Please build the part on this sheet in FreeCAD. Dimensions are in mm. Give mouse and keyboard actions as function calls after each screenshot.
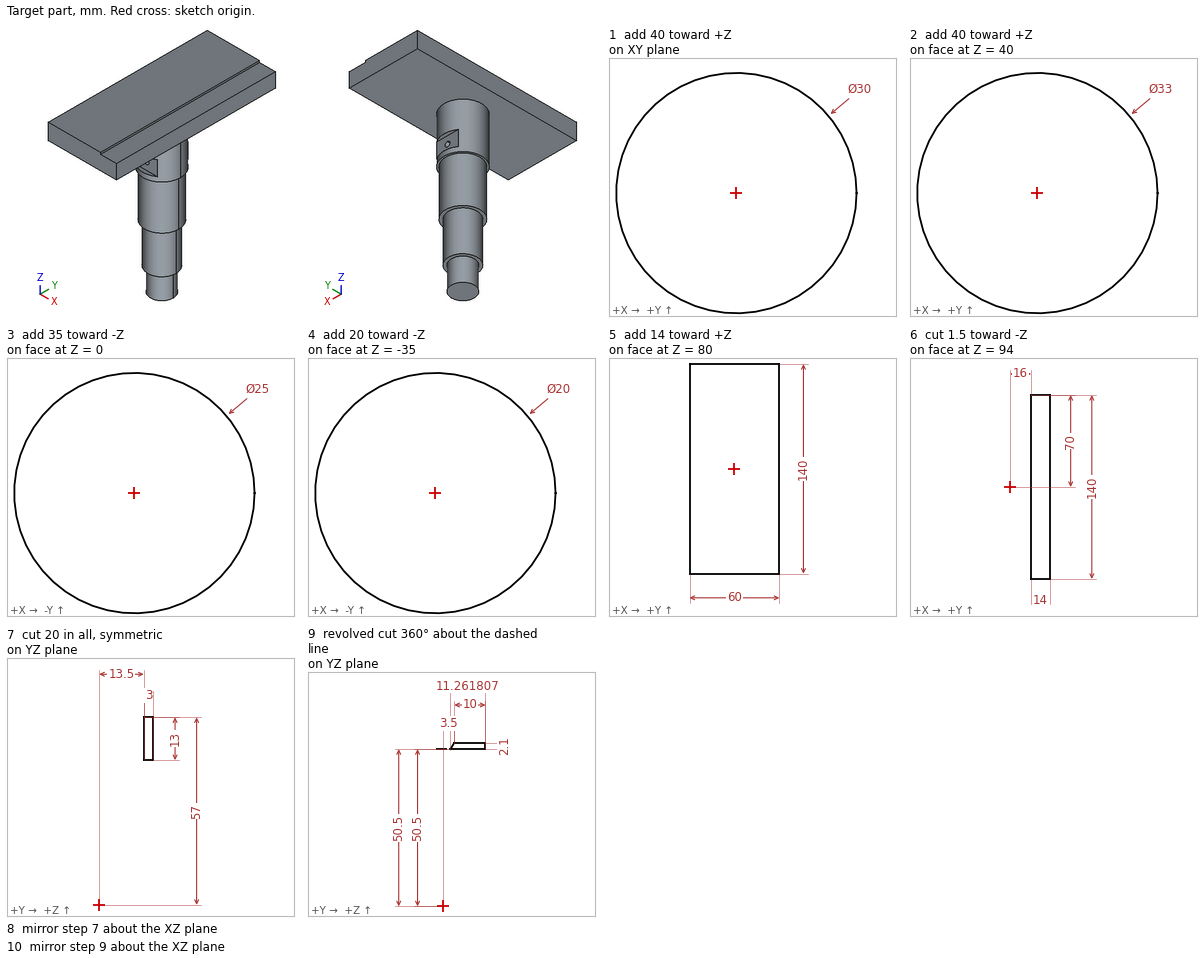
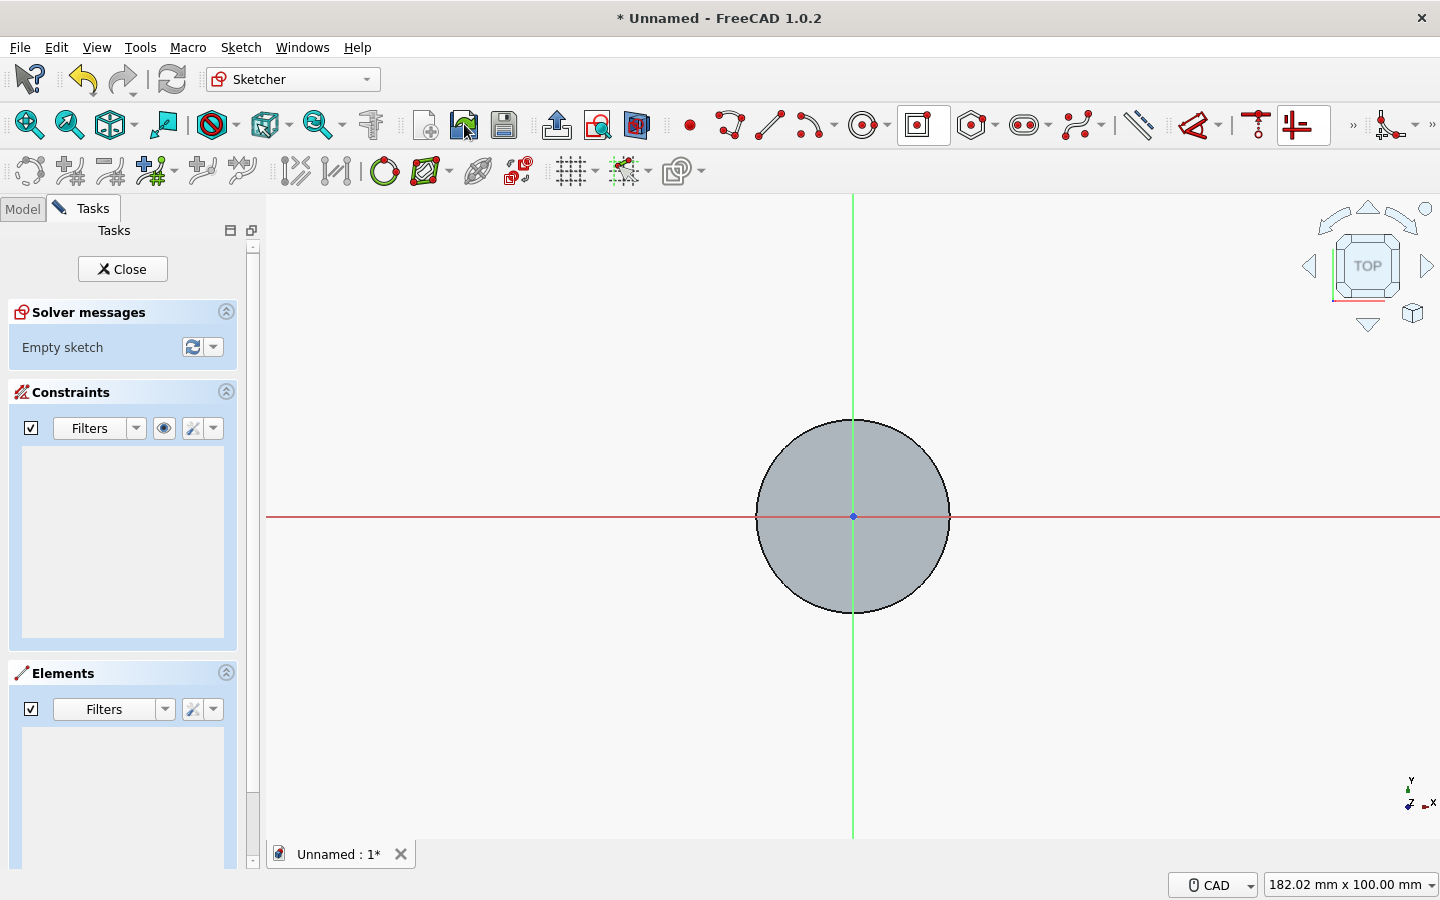
scroll(936, 516, up, 3)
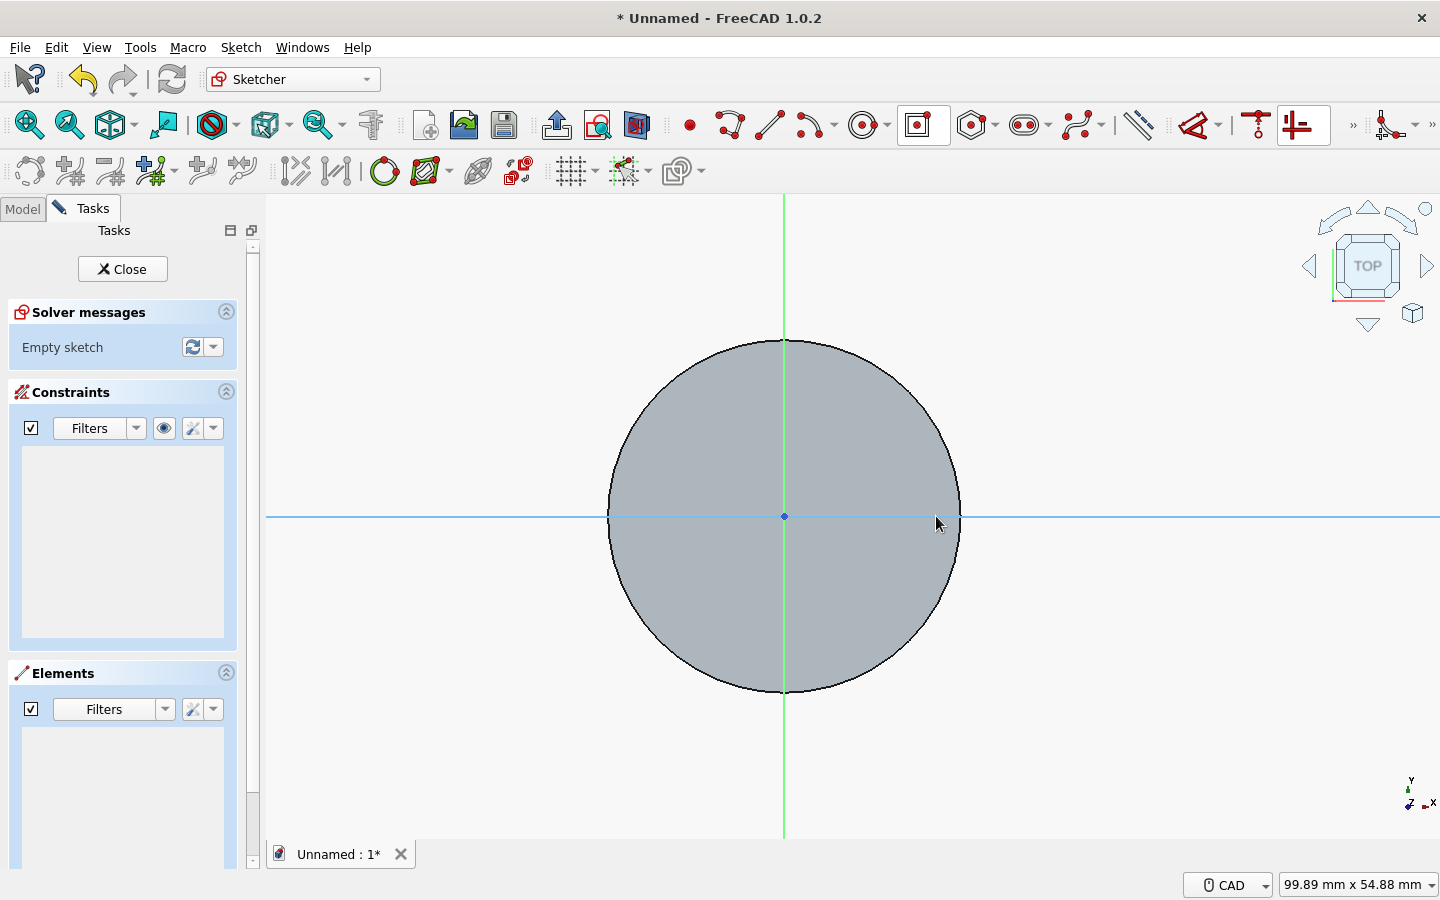
click(864, 126)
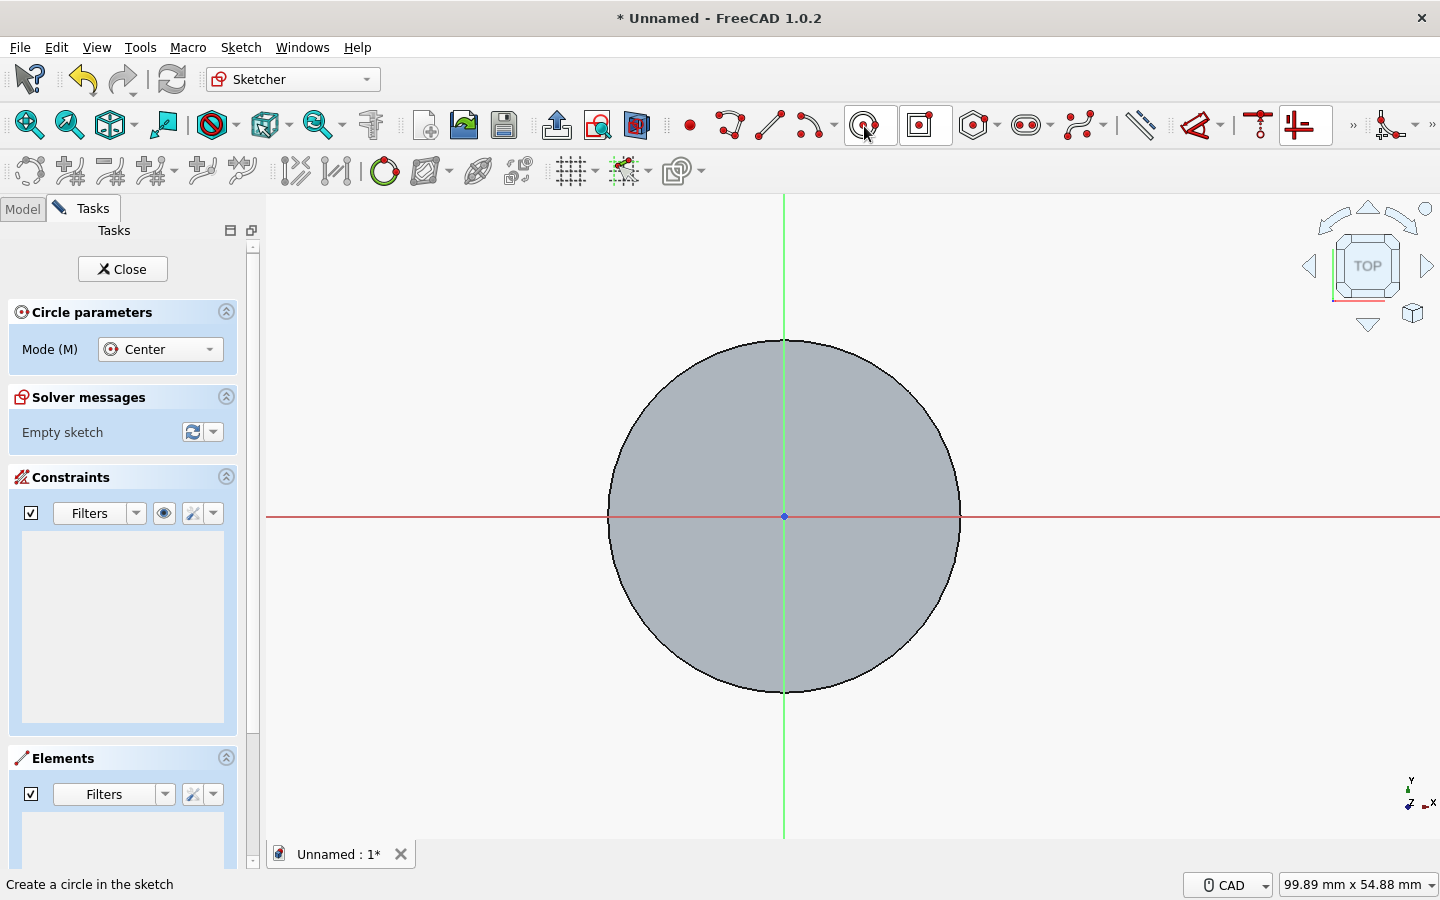
click(784, 516)
move(921, 379)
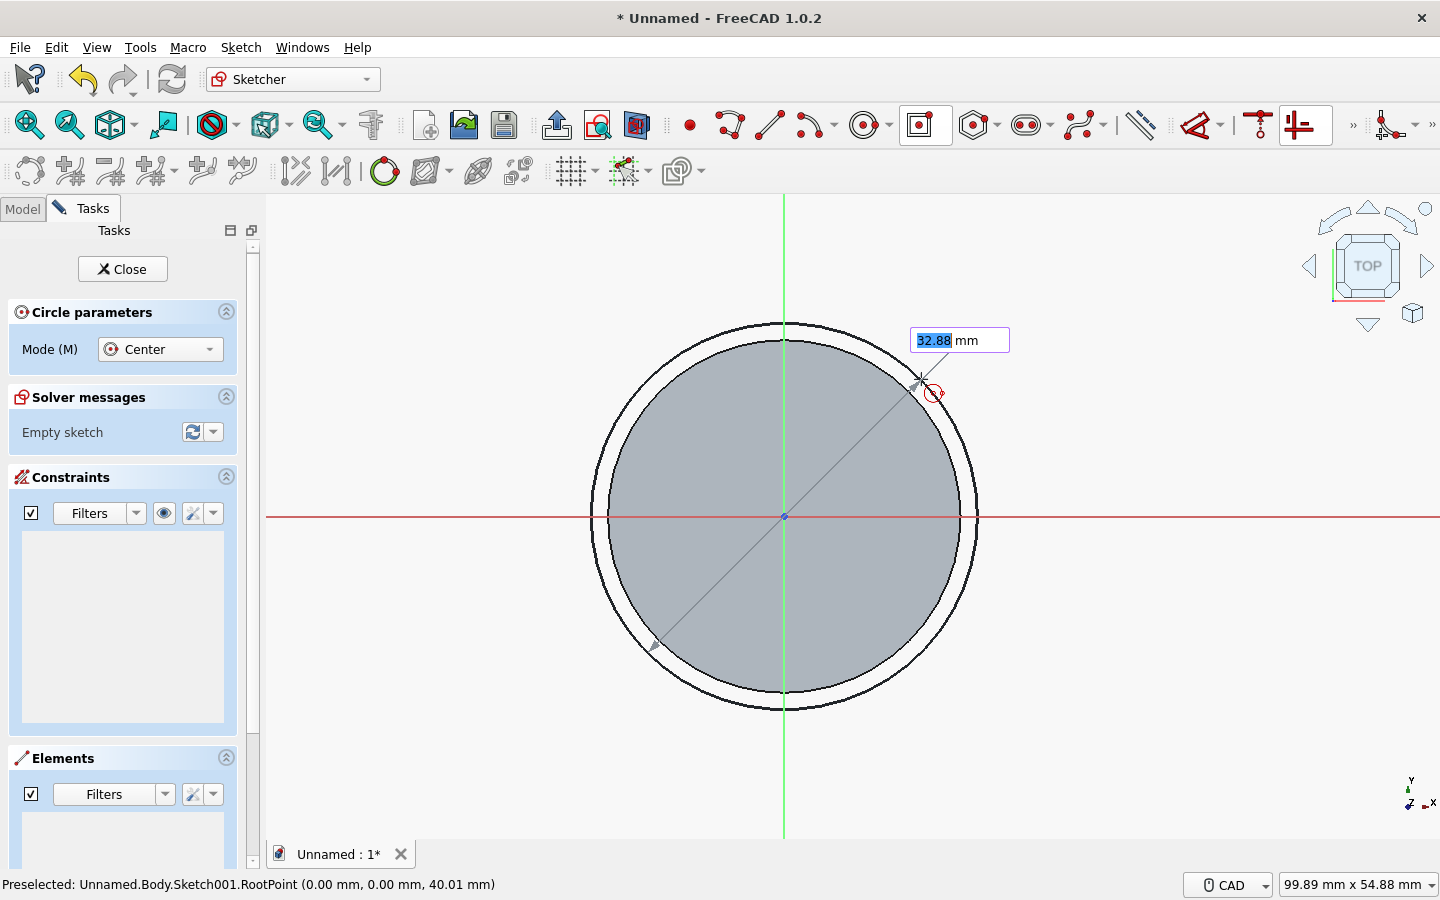
text(33)
key(Return)
key(Escape)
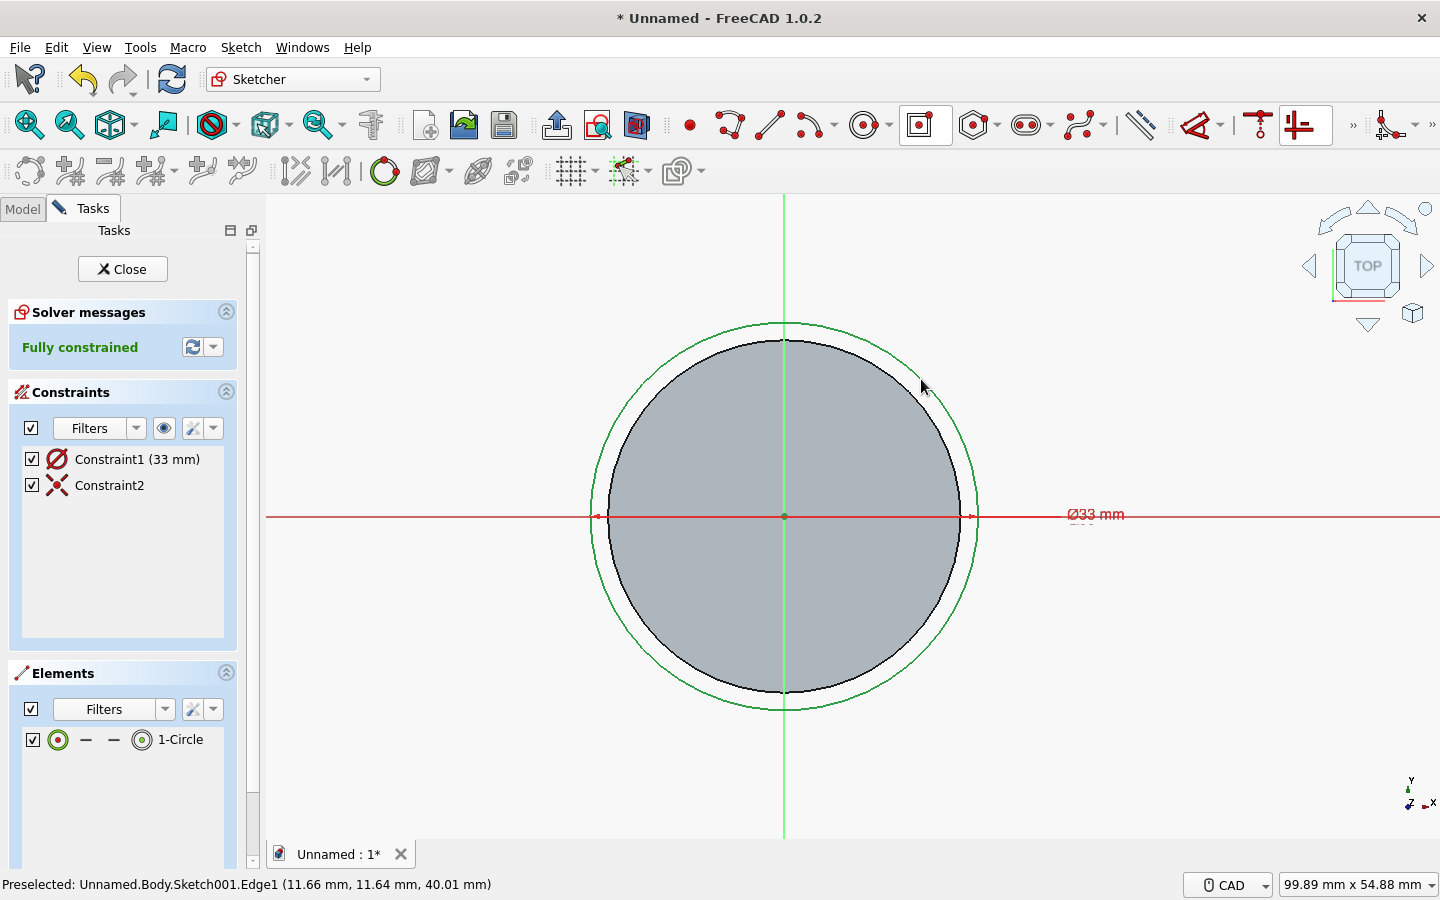
click(123, 269)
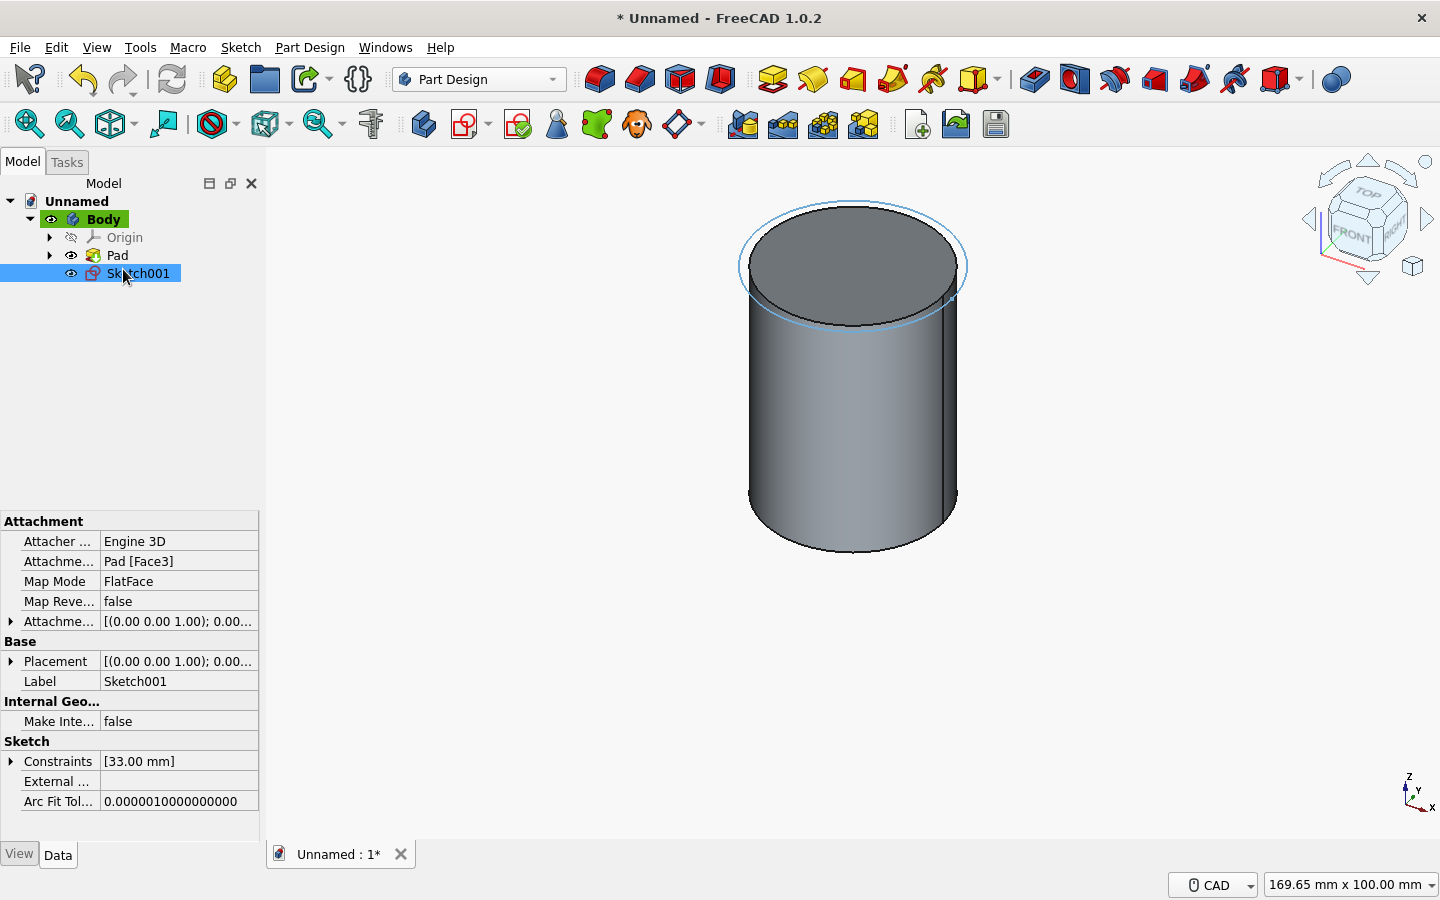
click(774, 80)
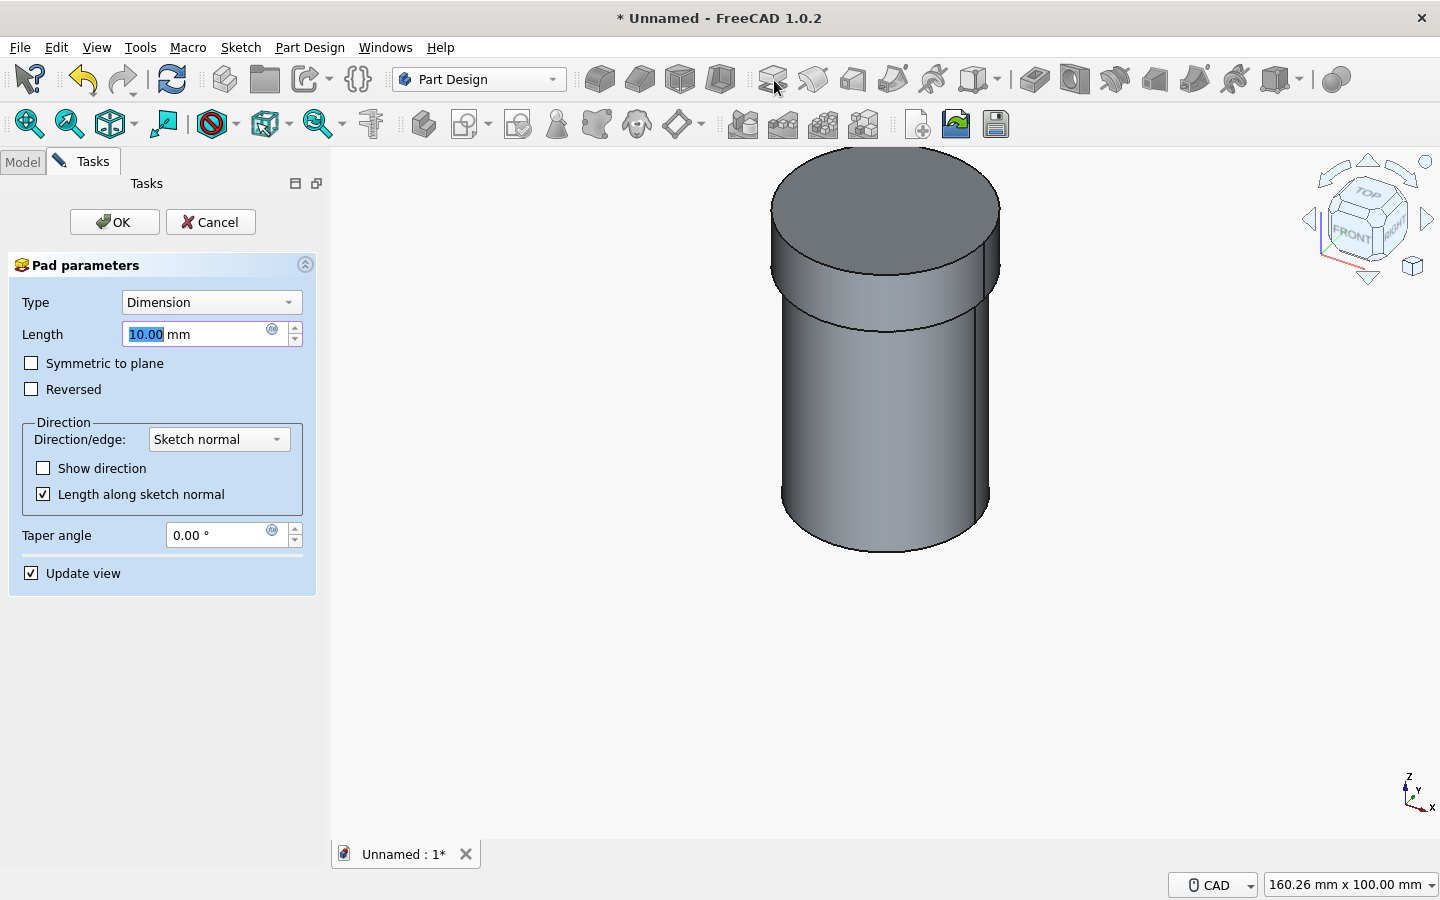
text(40)
key(Tab)